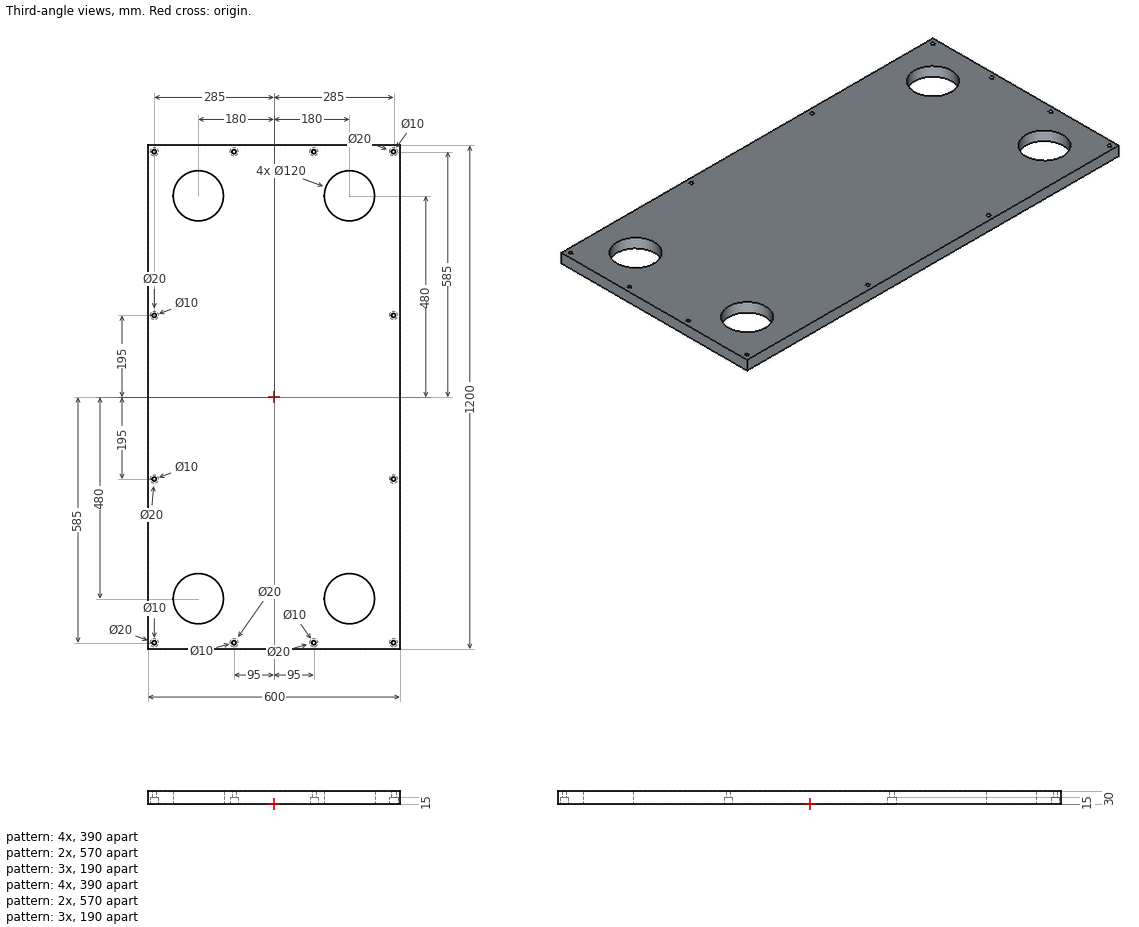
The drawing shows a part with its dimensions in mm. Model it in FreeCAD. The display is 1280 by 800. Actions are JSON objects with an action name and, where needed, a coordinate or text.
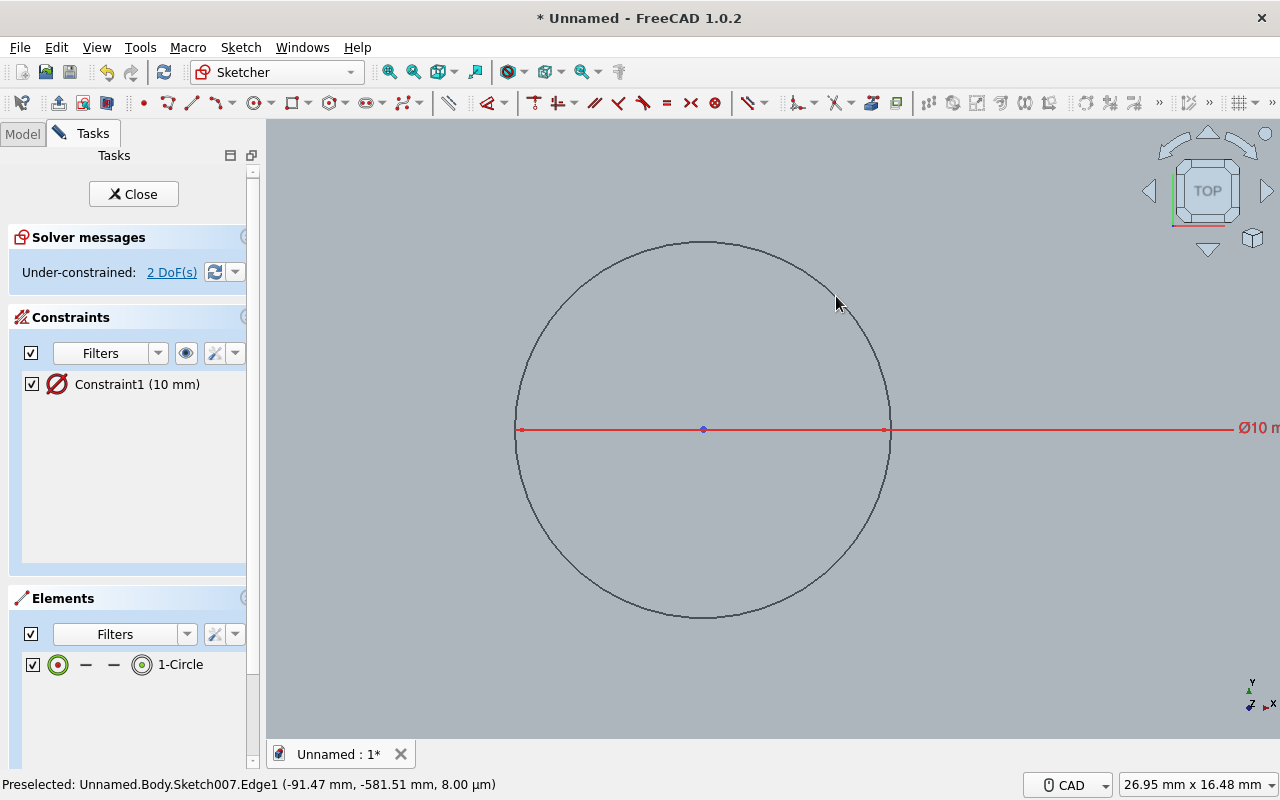
{"action": "key", "text": "d"}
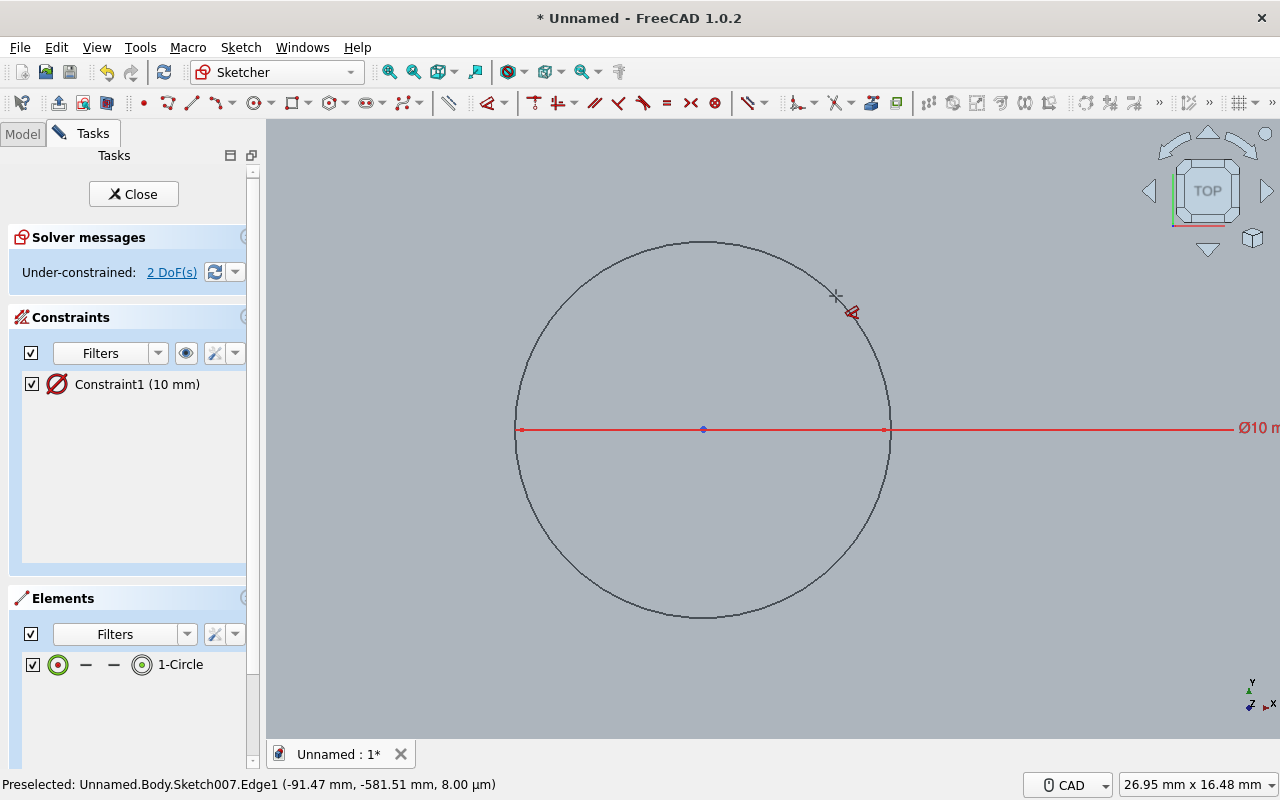
{"action": "left_click", "coordinate": [703, 430]}
{"action": "left_click", "coordinate": [909, 464]}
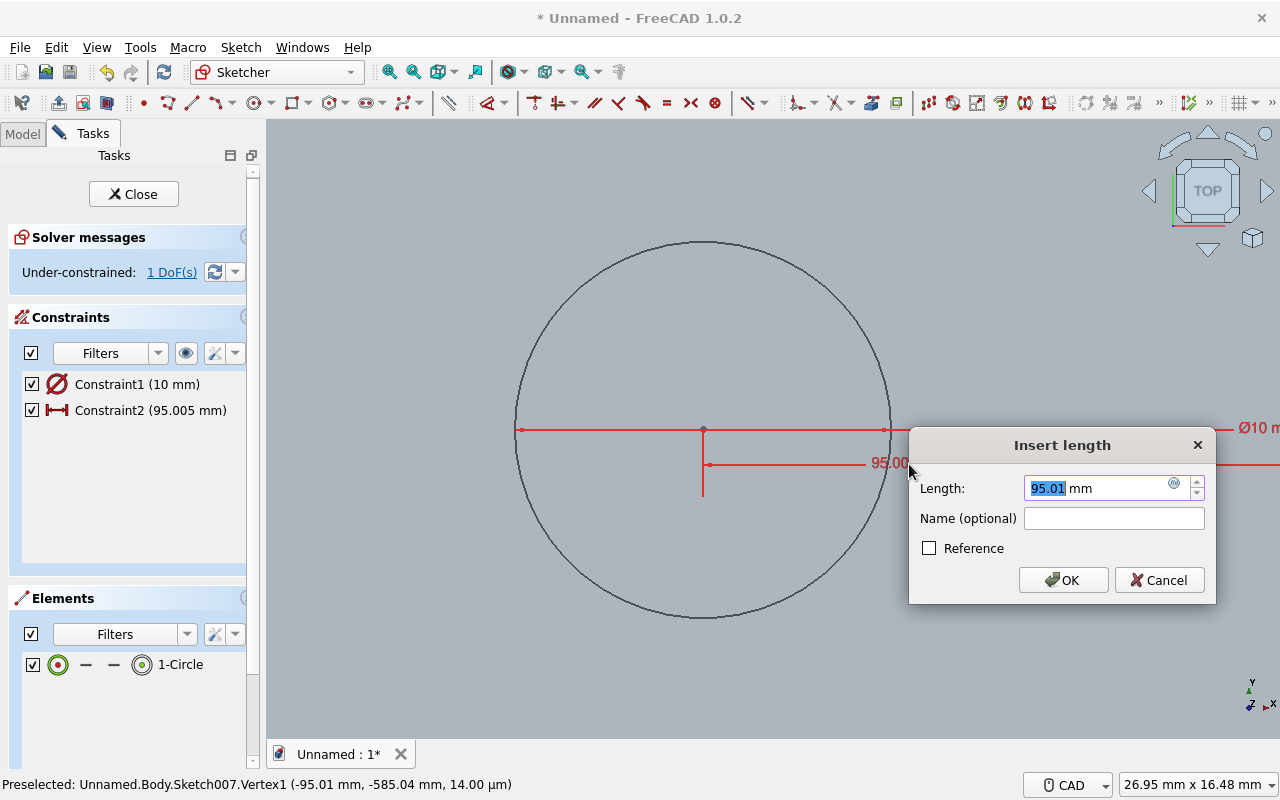
{"action": "type", "text": "95"}
{"action": "key", "text": "Return"}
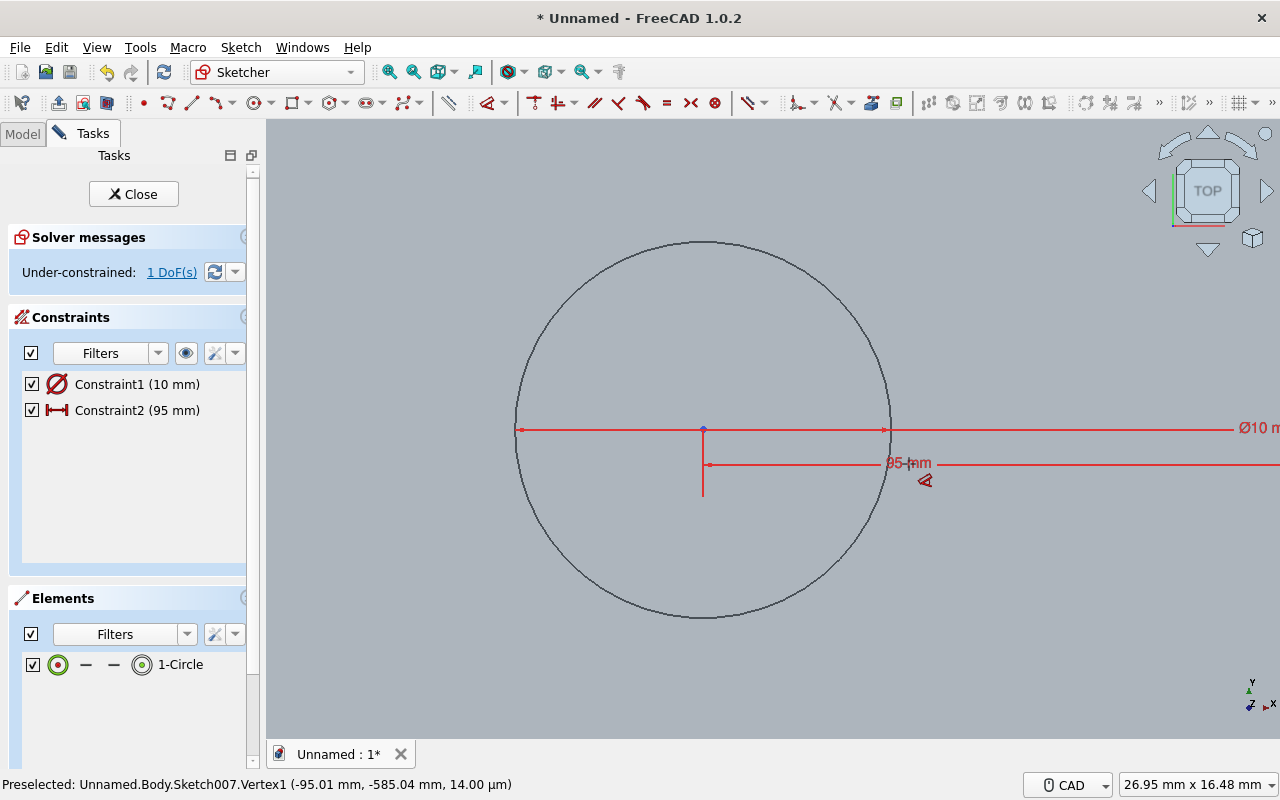
{"action": "left_click", "coordinate": [703, 430]}
{"action": "left_click", "coordinate": [669, 288]}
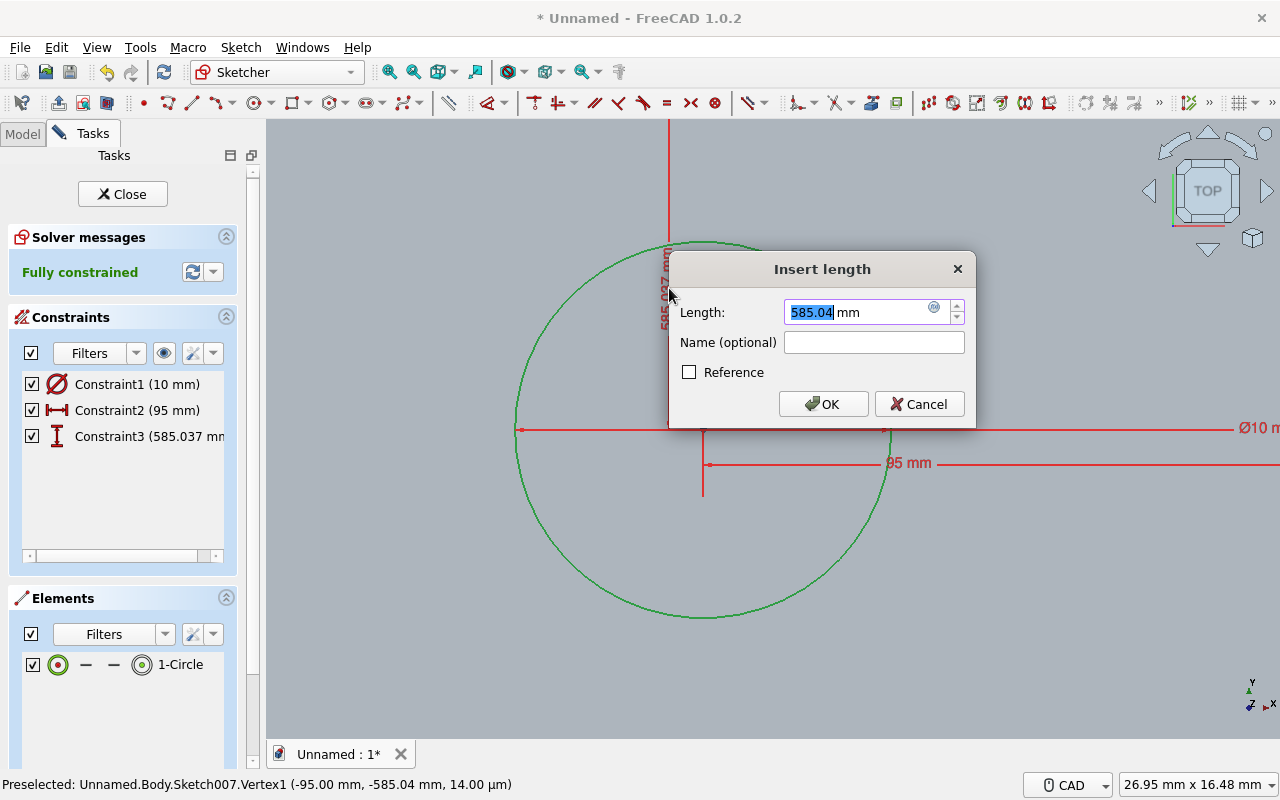
{"action": "type", "text": "585"}
{"action": "key", "text": "Return"}
{"action": "key", "text": "Escape"}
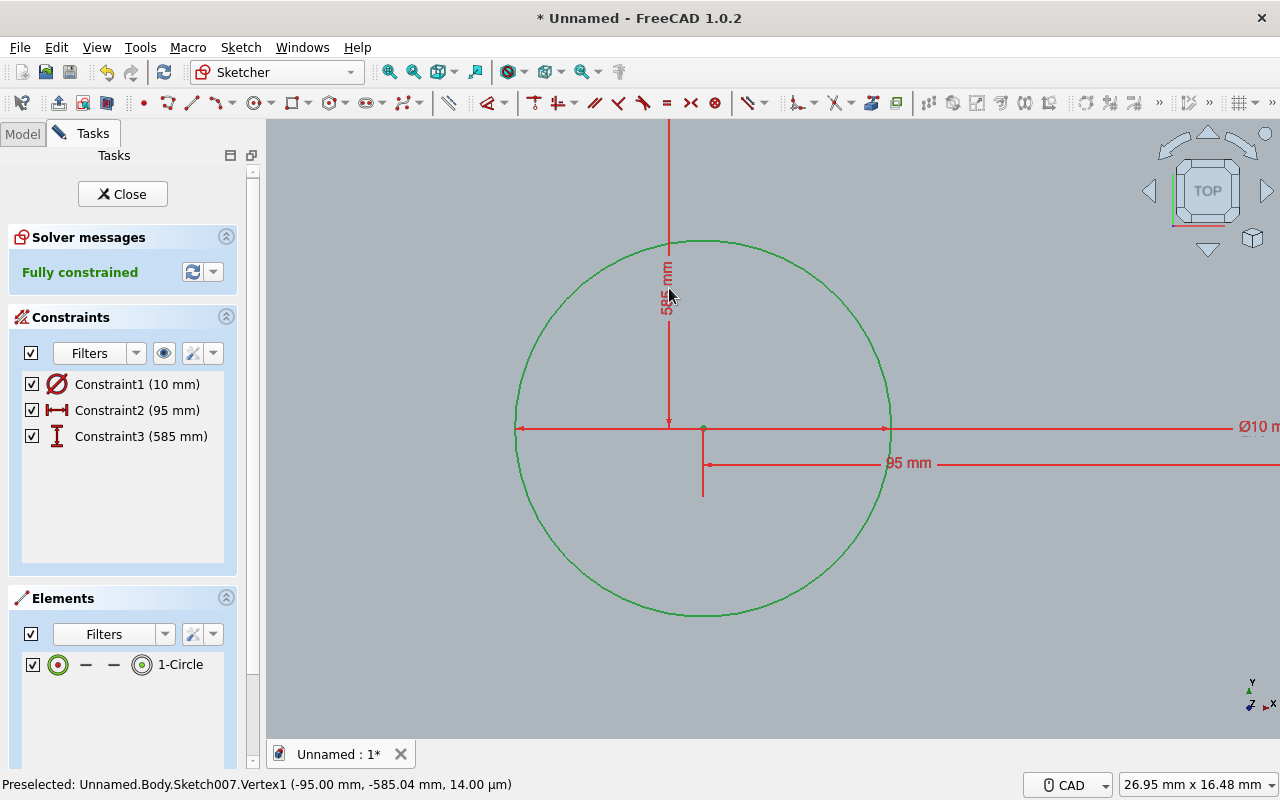
{"action": "left_click", "coordinate": [123, 194]}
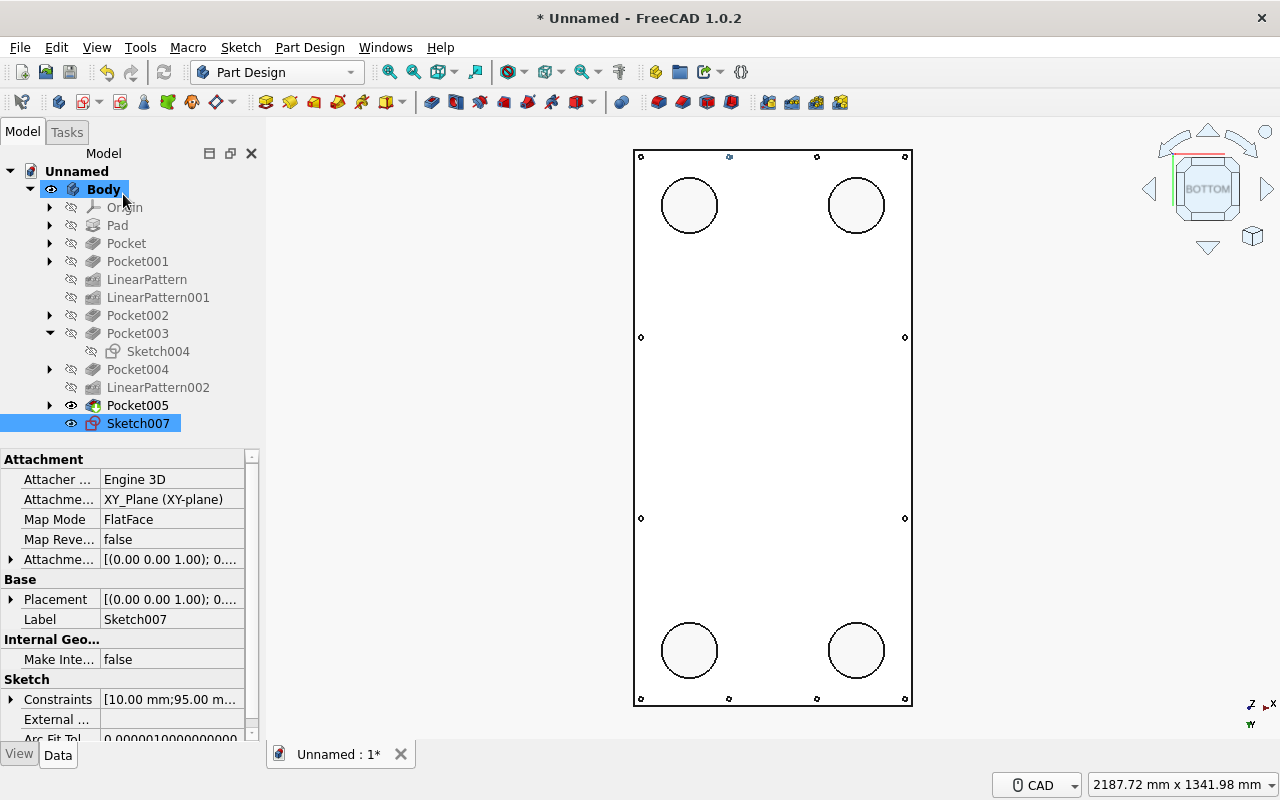
{"action": "left_click", "coordinate": [432, 102]}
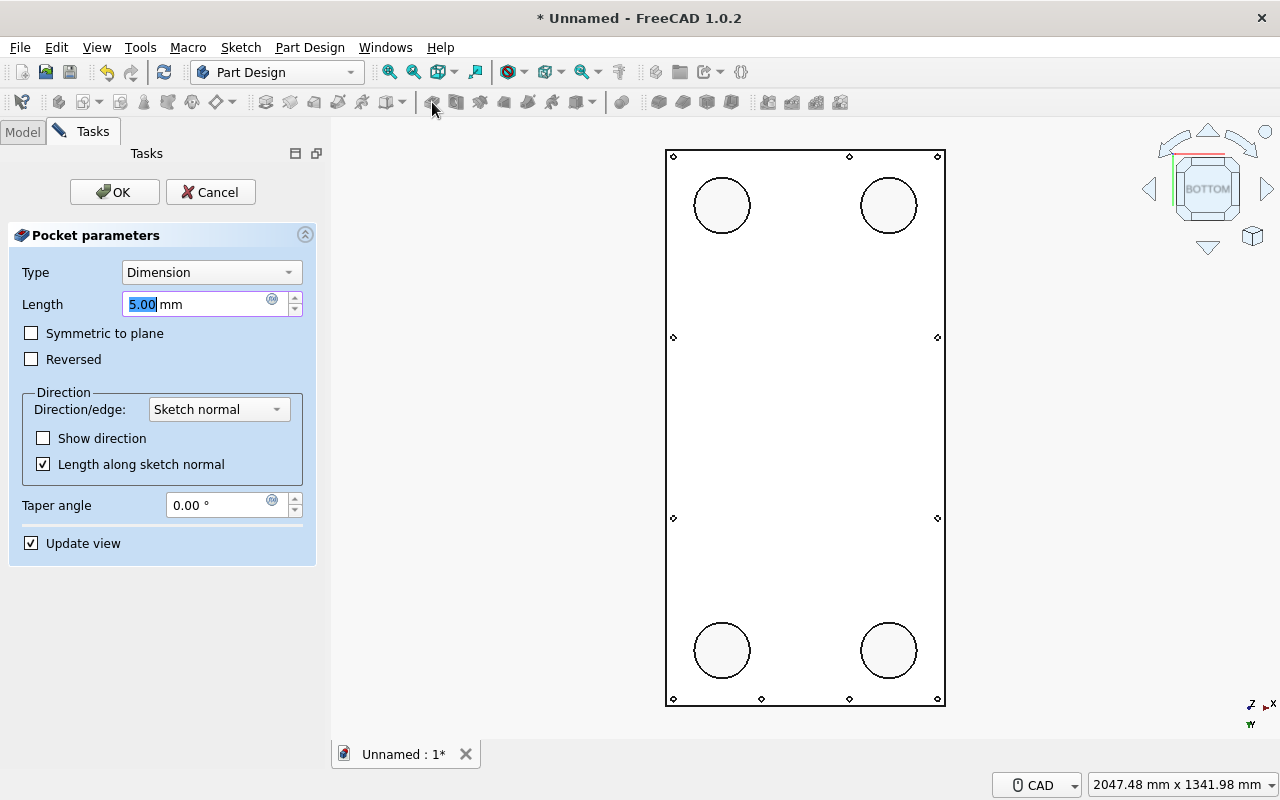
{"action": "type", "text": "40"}
{"action": "key", "text": "Tab"}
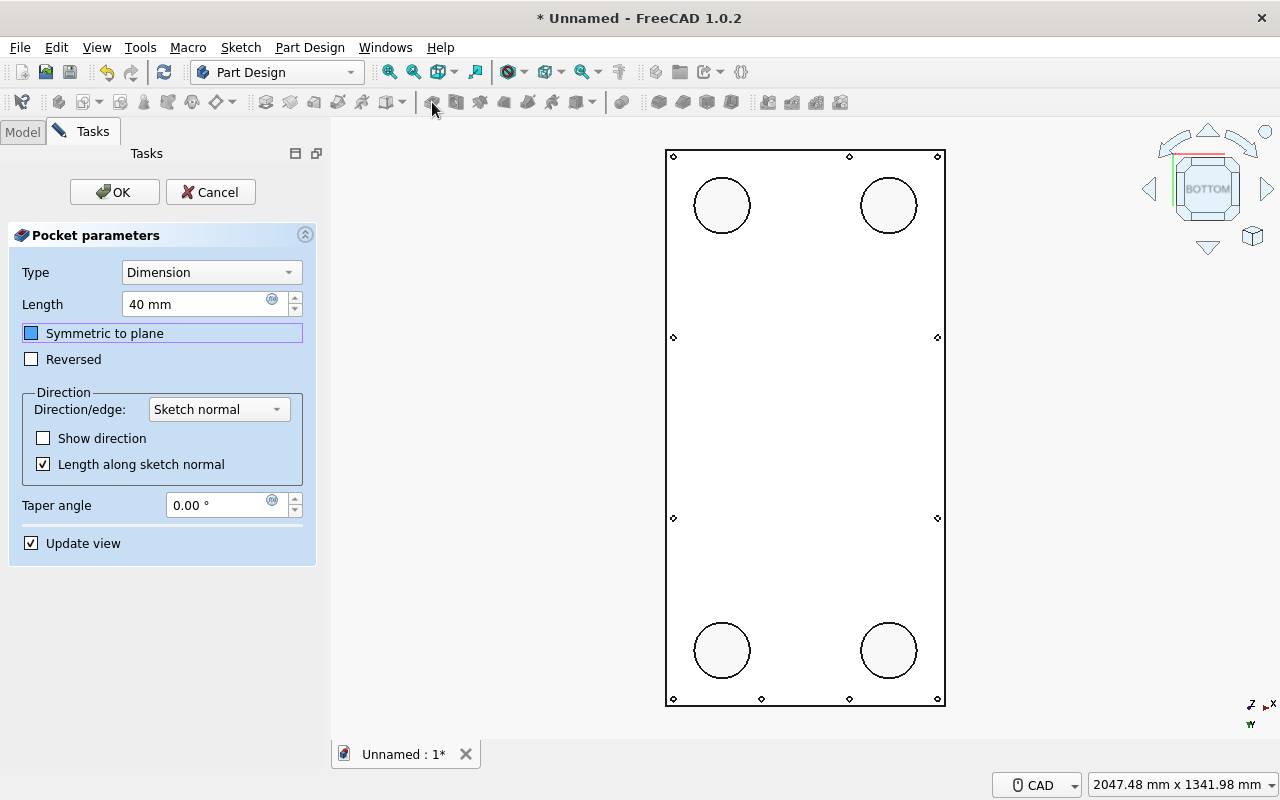
{"action": "left_click", "coordinate": [30, 359]}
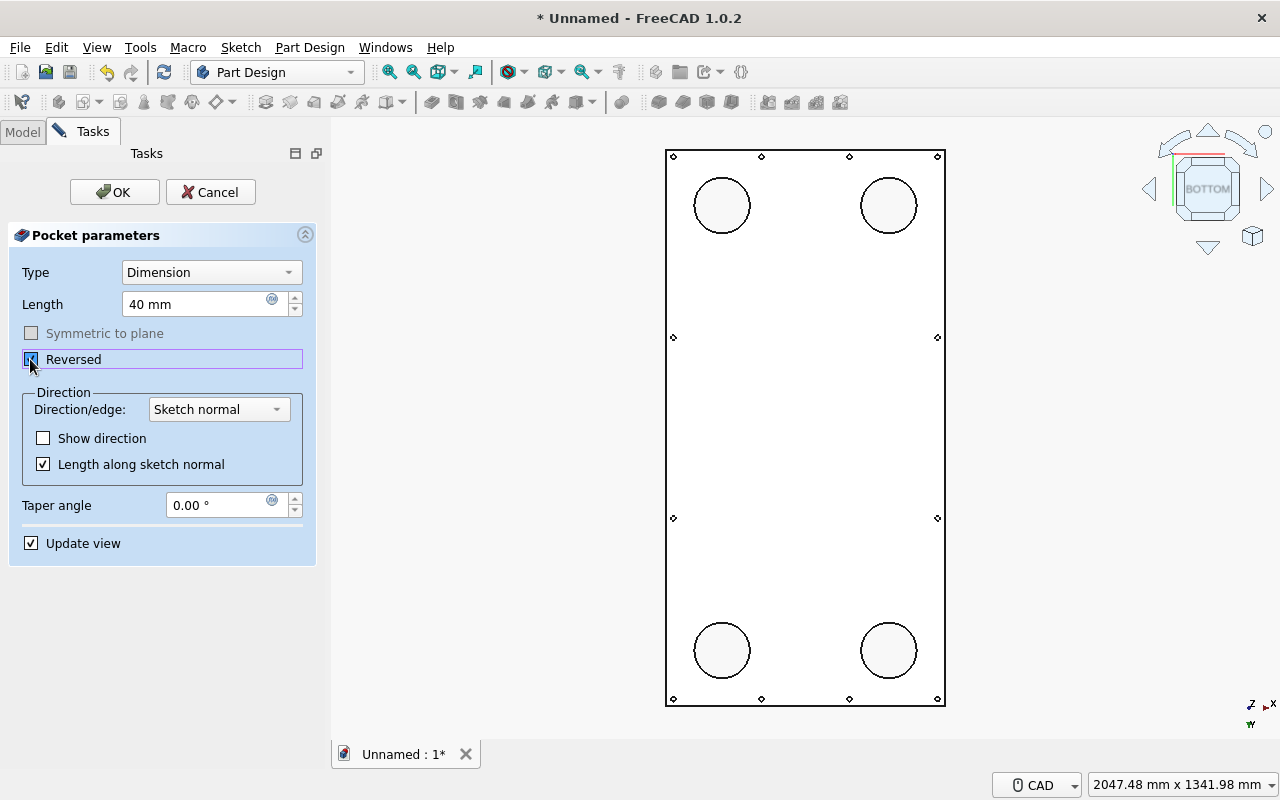
{"action": "left_click", "coordinate": [115, 192]}